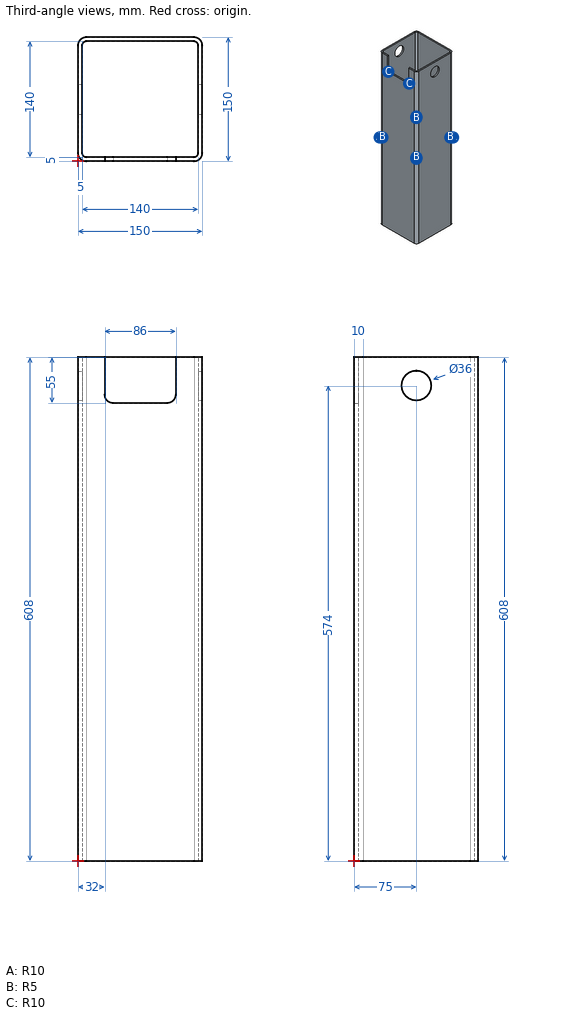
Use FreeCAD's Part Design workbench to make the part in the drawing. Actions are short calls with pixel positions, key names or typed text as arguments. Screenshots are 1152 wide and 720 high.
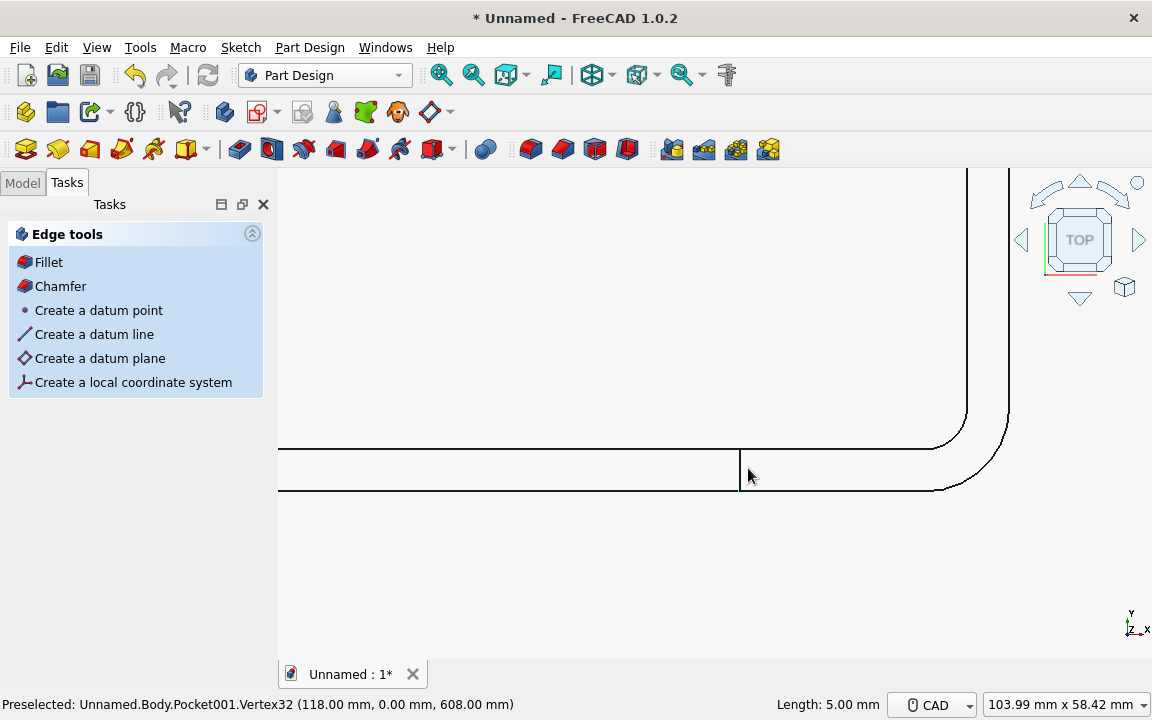
key(v)
key(f)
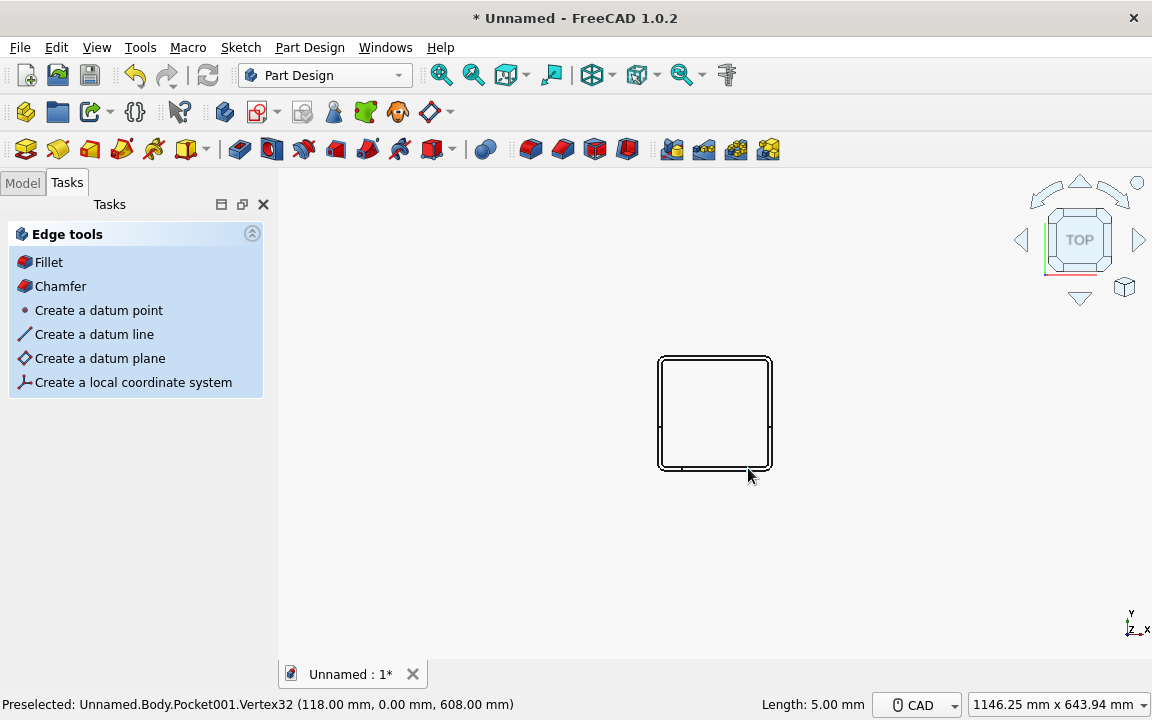
key(1)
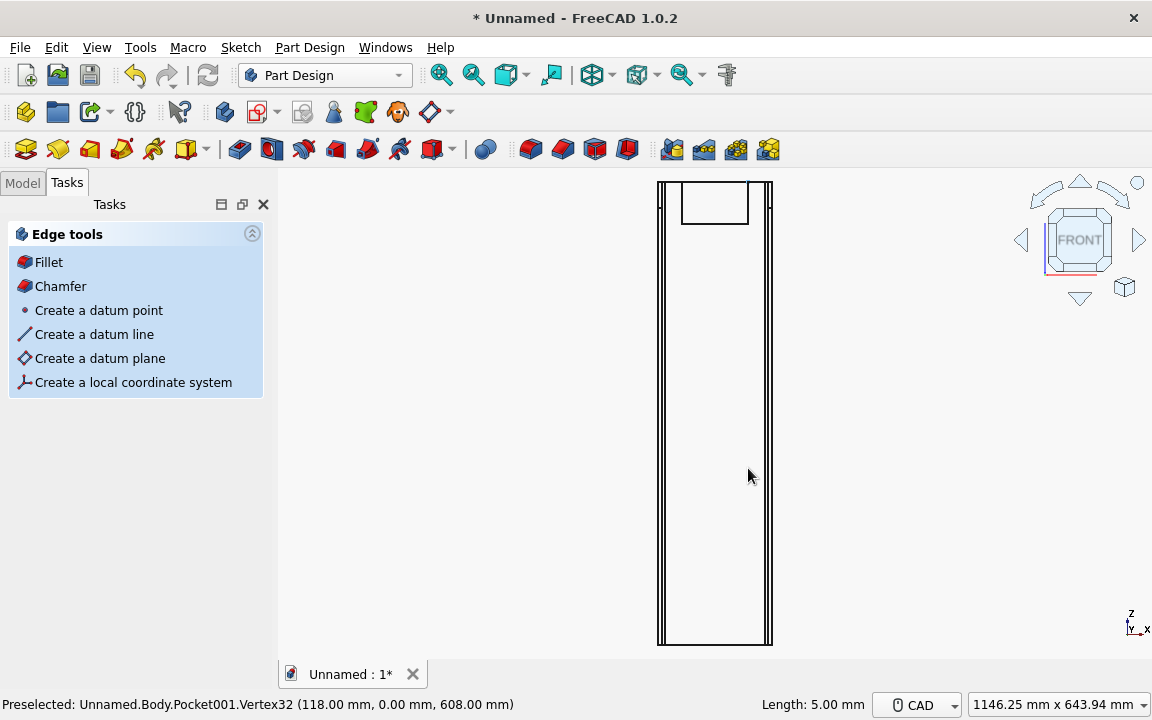
scroll(748, 223, up, 12)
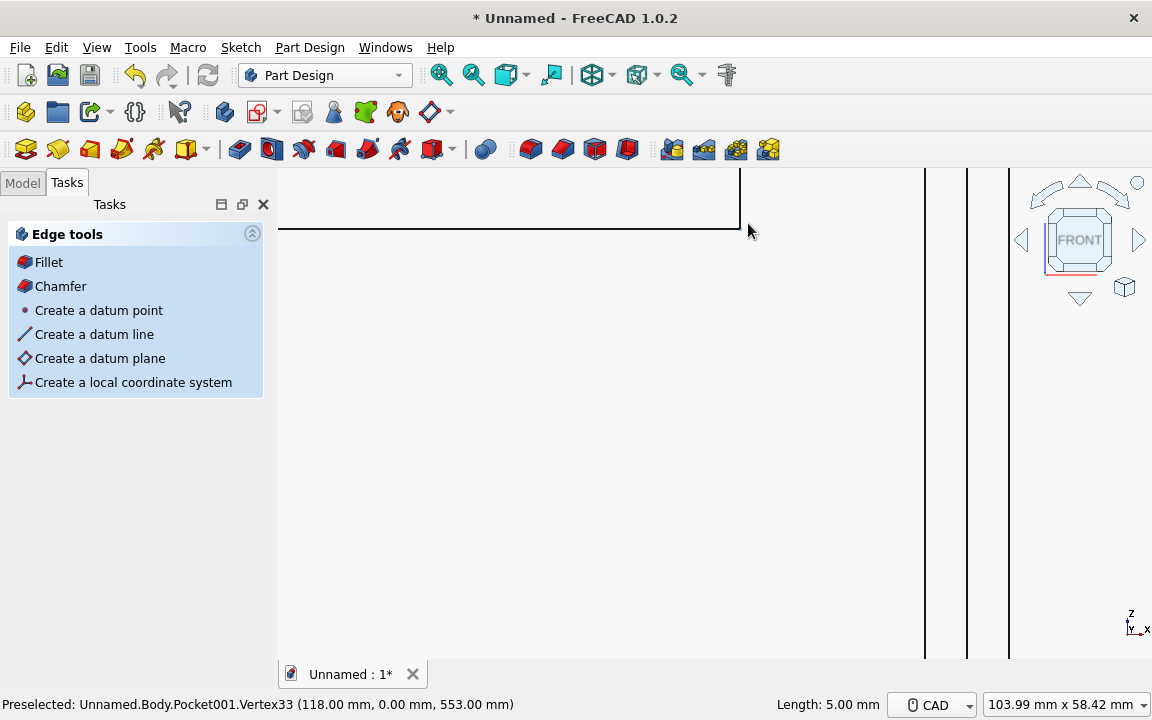
key(v)
key(f)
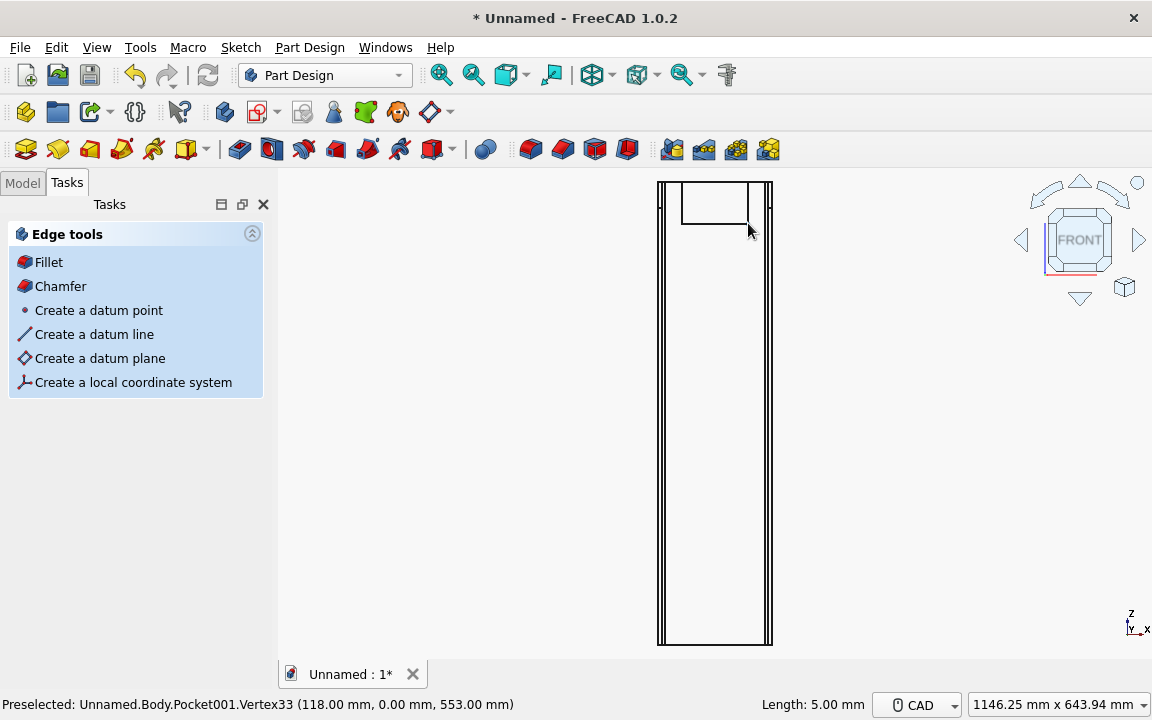
key(3)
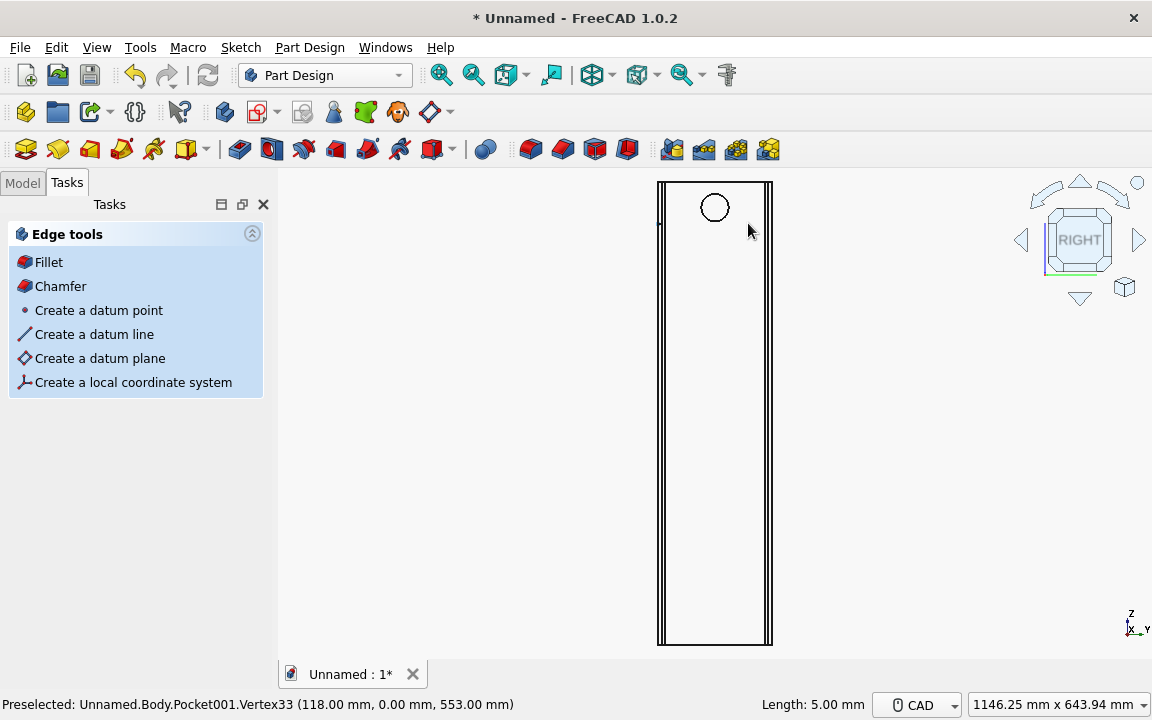
scroll(660, 223, up, 12)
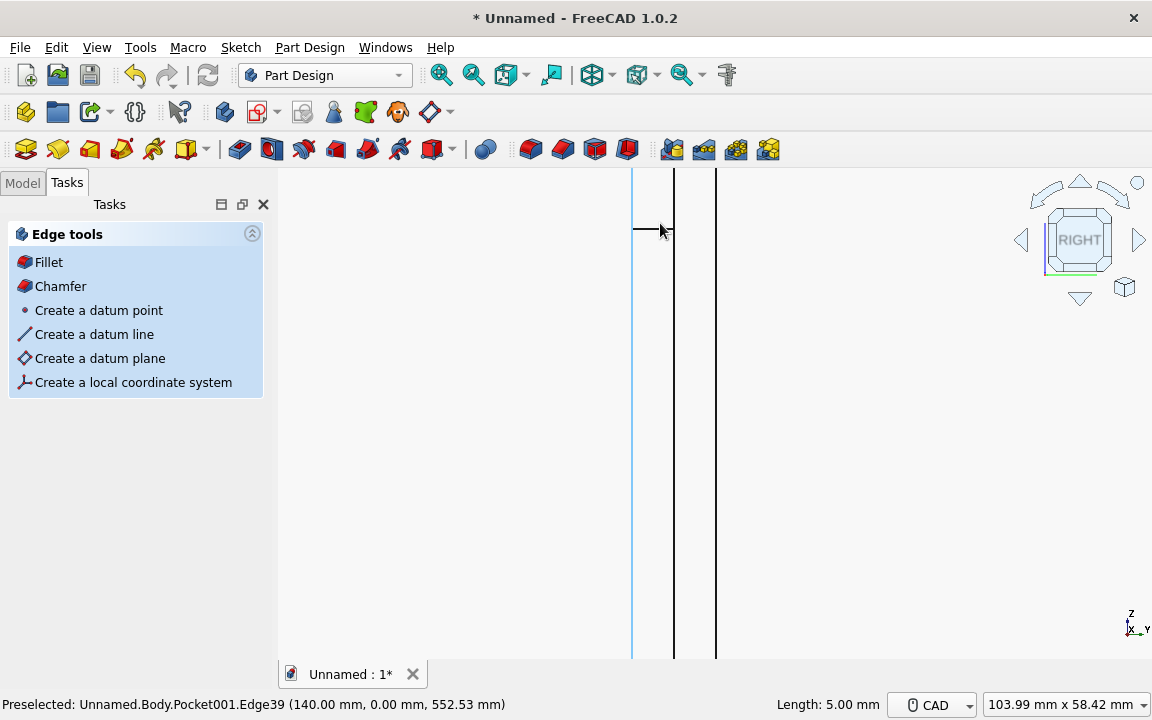
click(653, 228, ctrl)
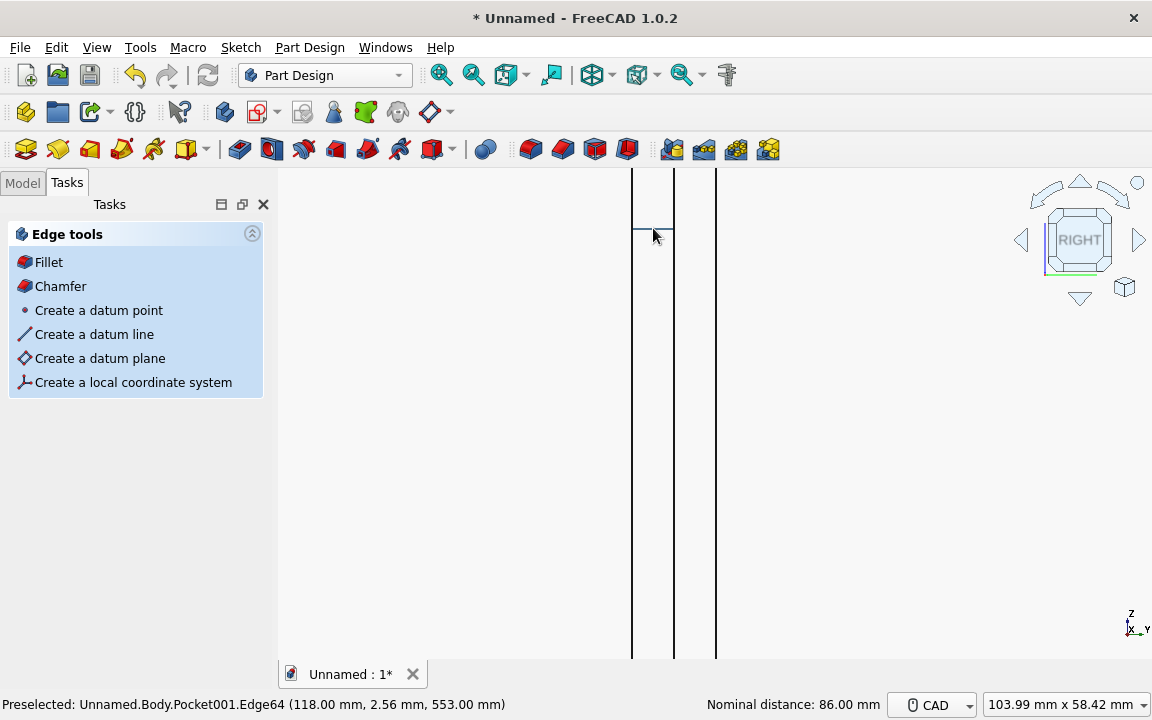
key(v)
key(1)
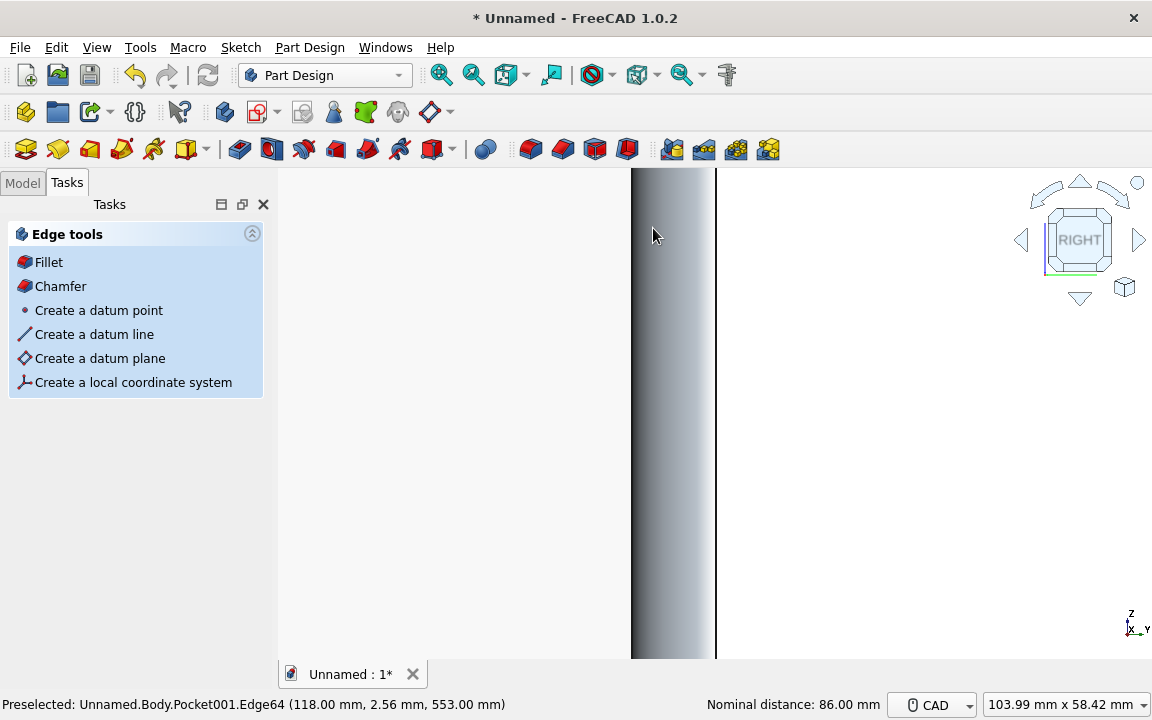
click(532, 150)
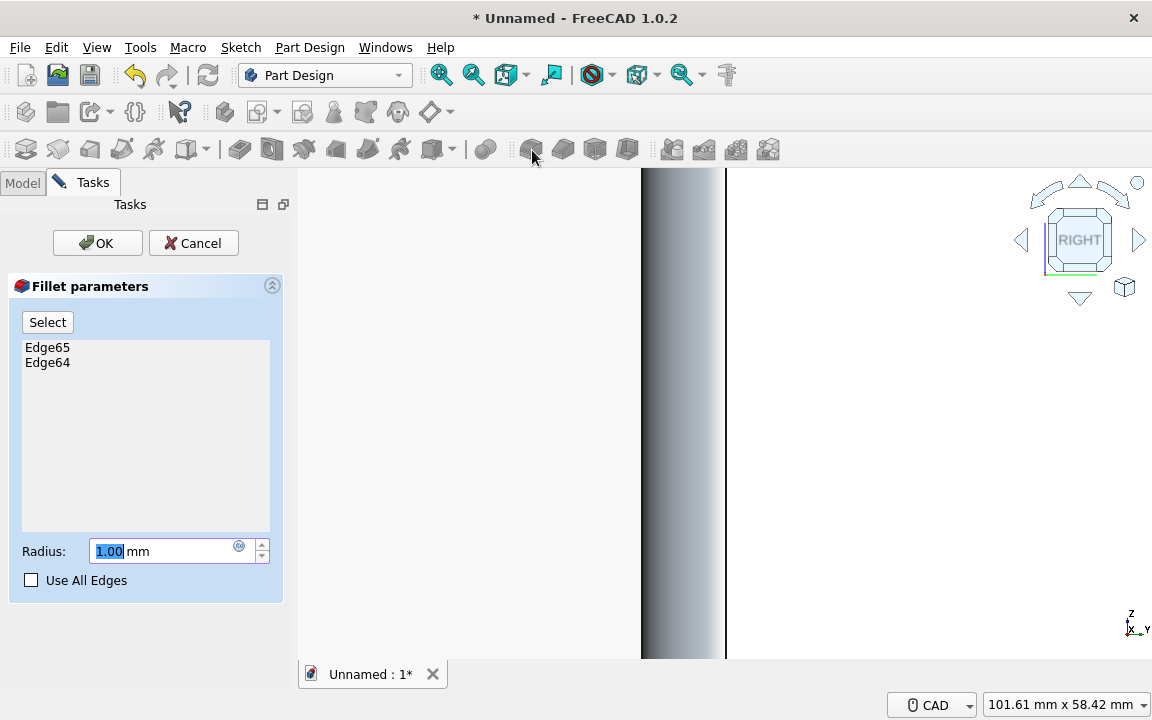
text(10)
key(Tab)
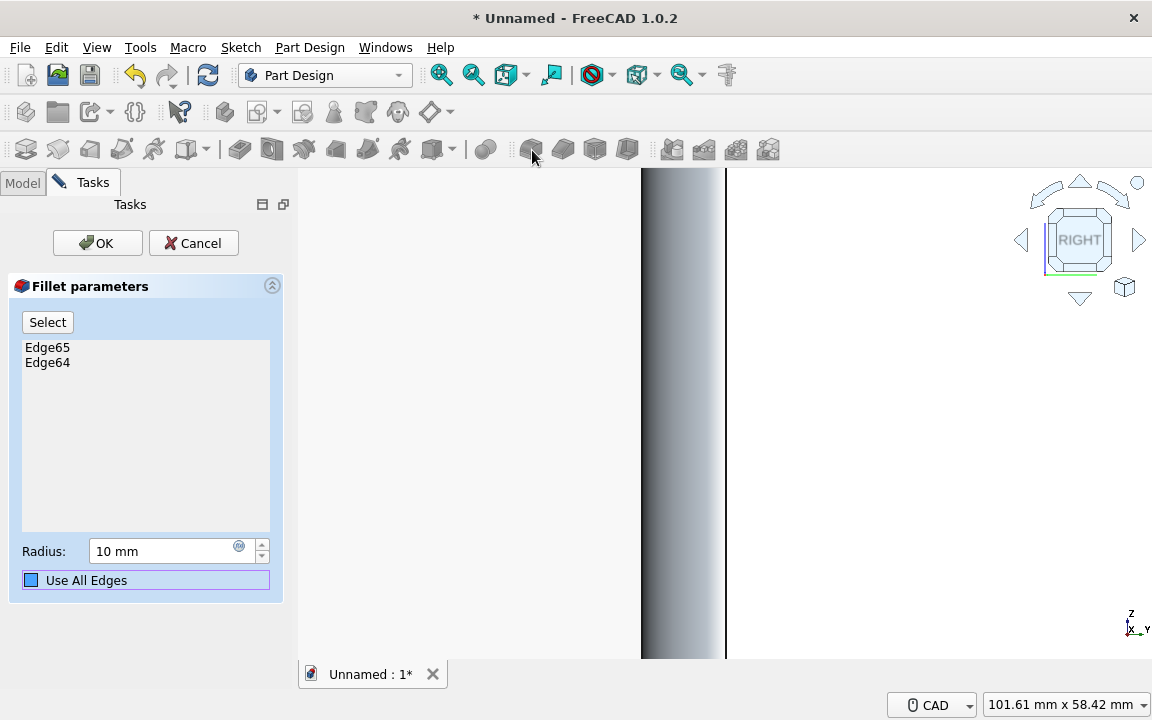
click(98, 243)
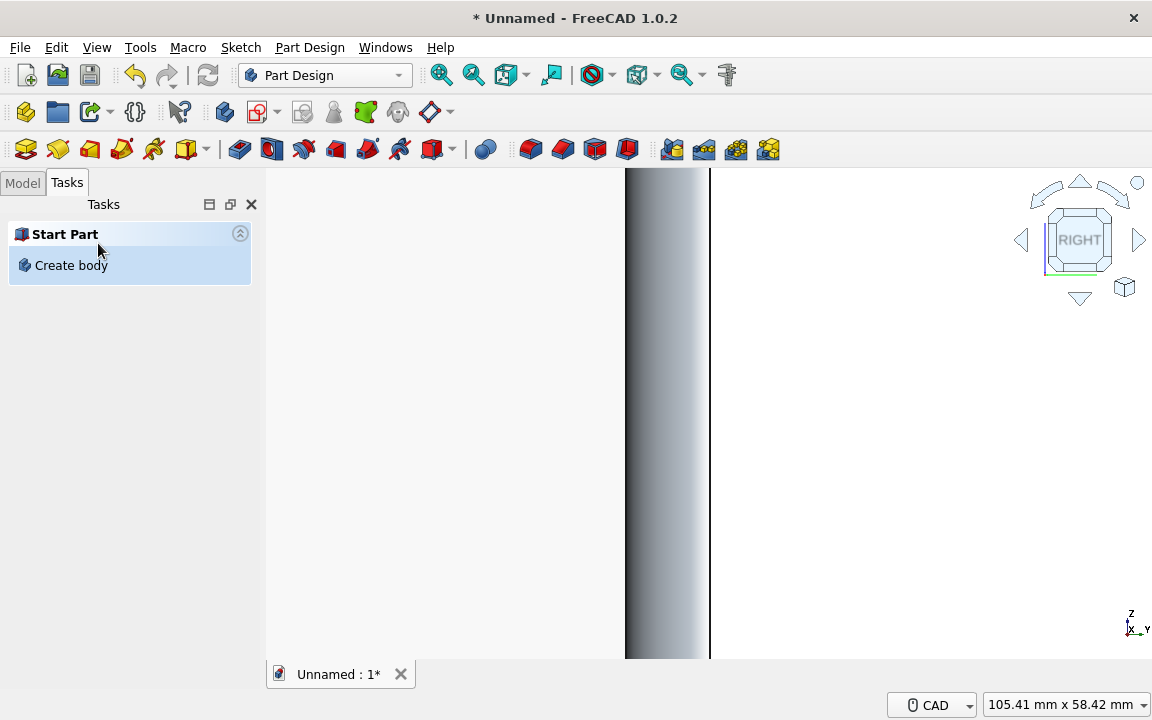
key(0)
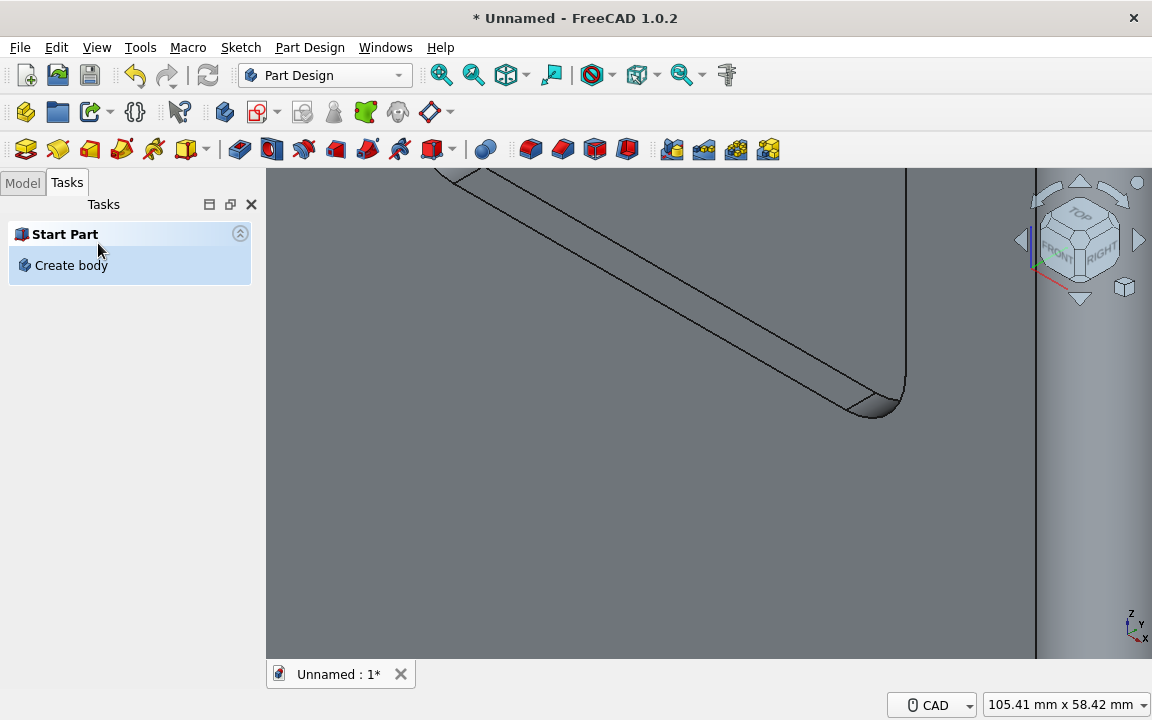
key(v)
key(f)